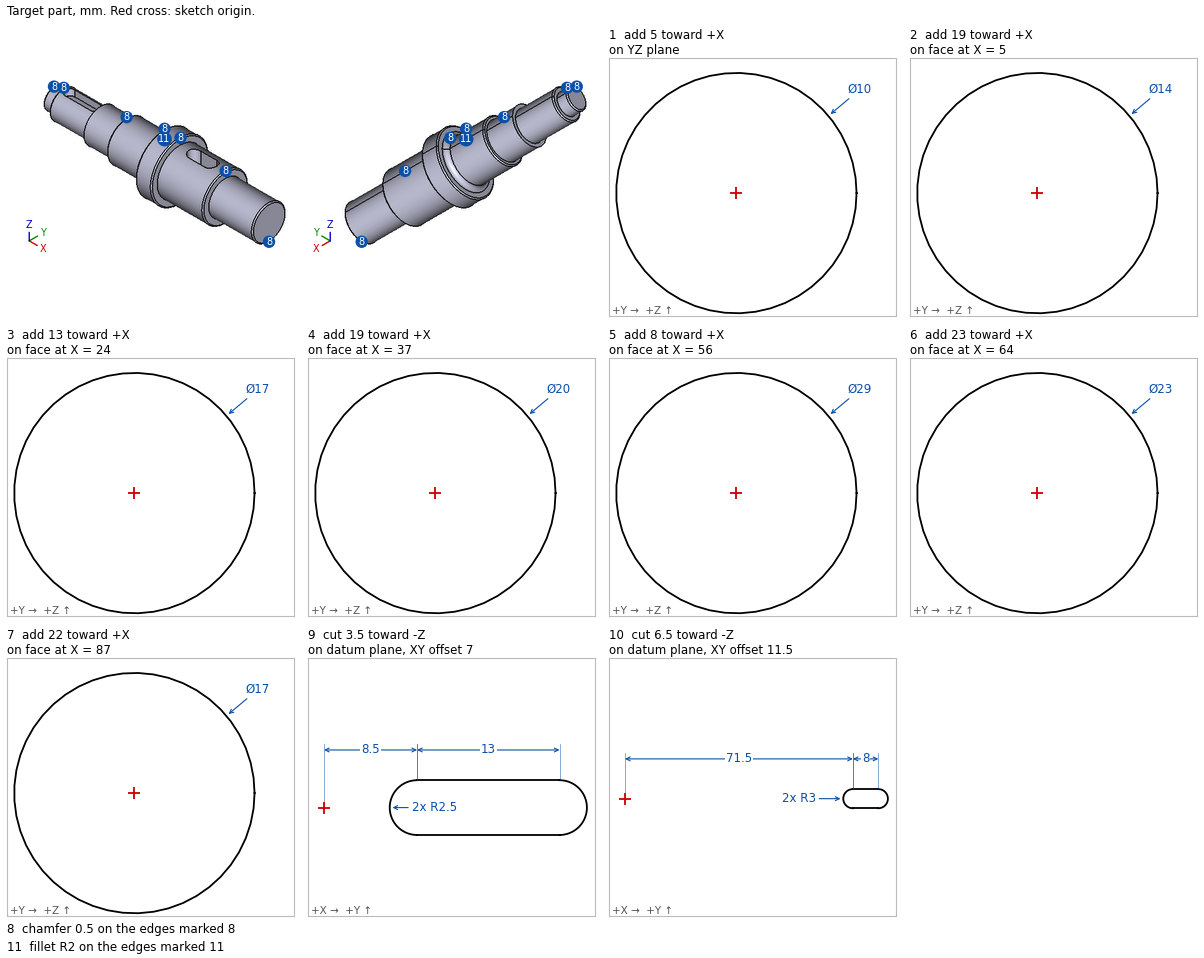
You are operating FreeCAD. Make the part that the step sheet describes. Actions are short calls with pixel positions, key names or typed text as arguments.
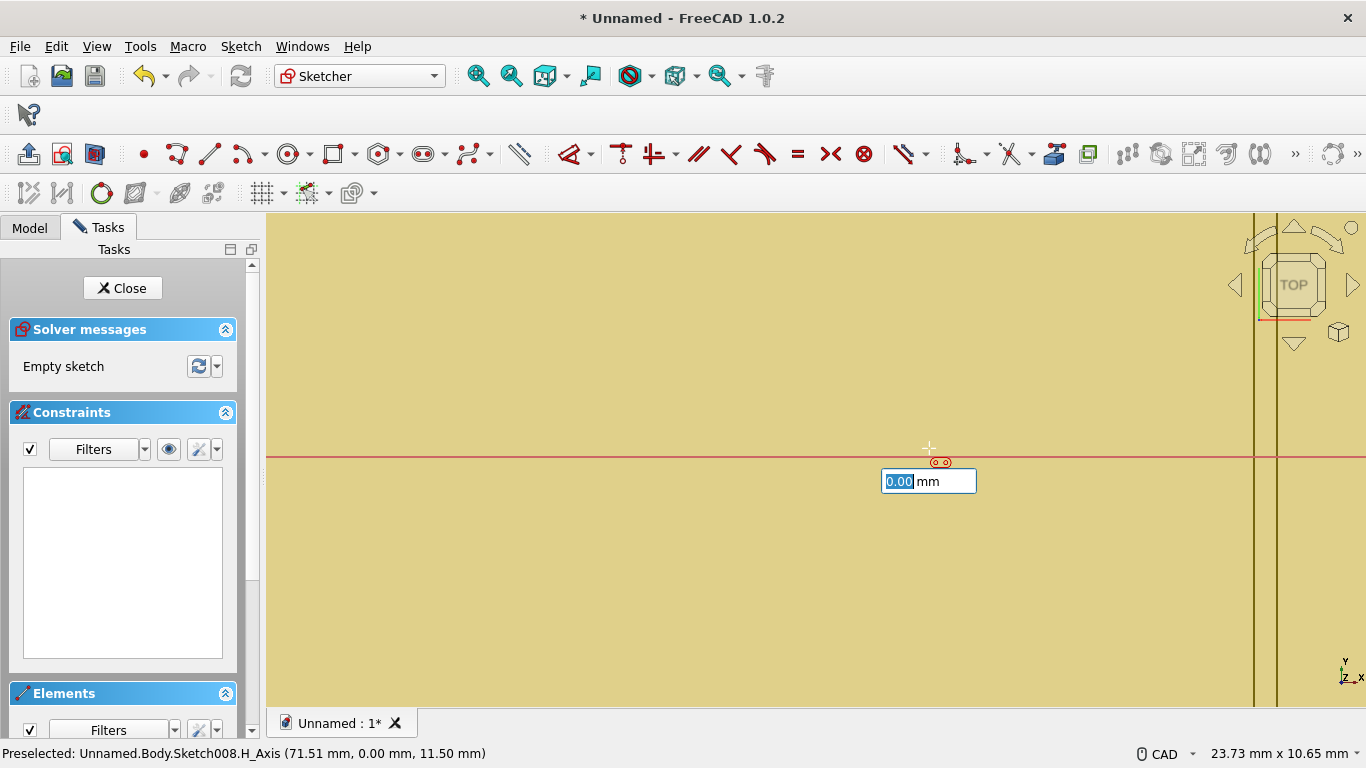
click(744, 317)
key(Escape)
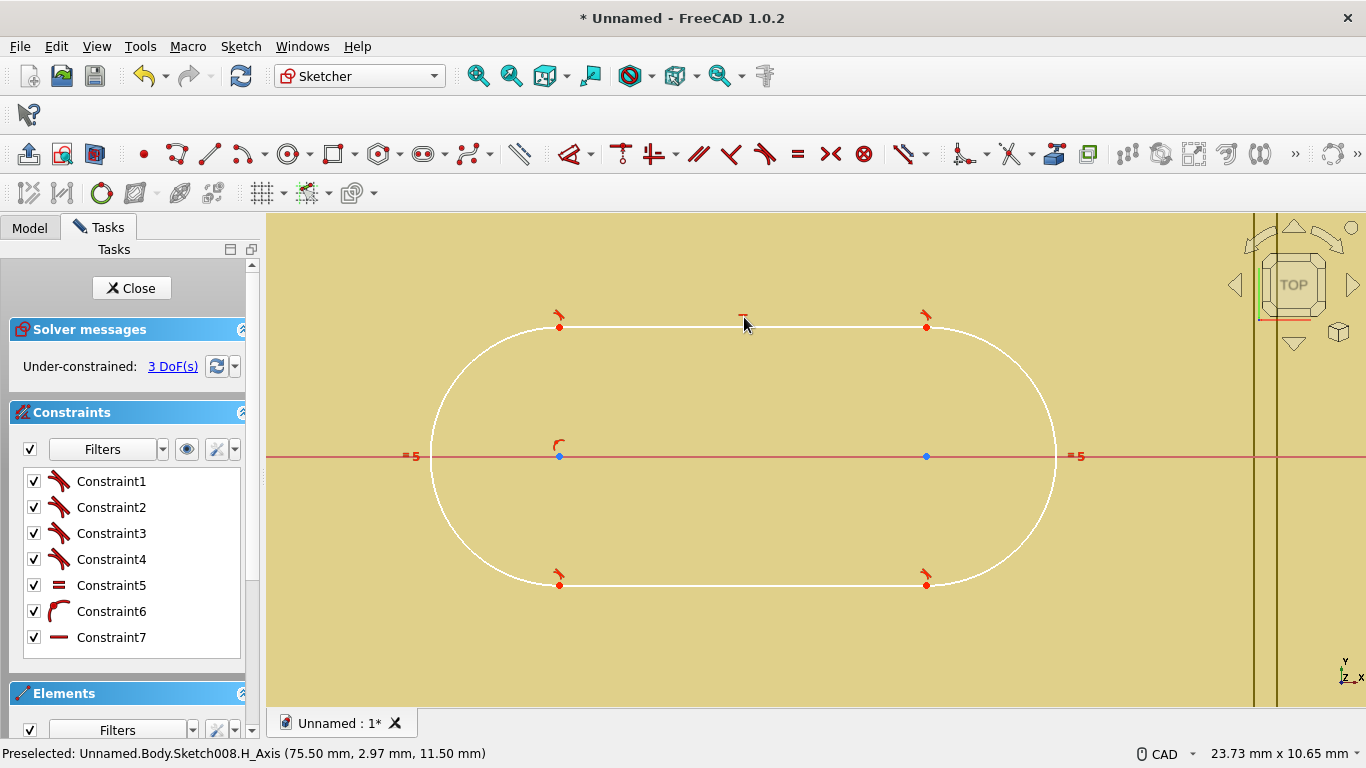
click(568, 154)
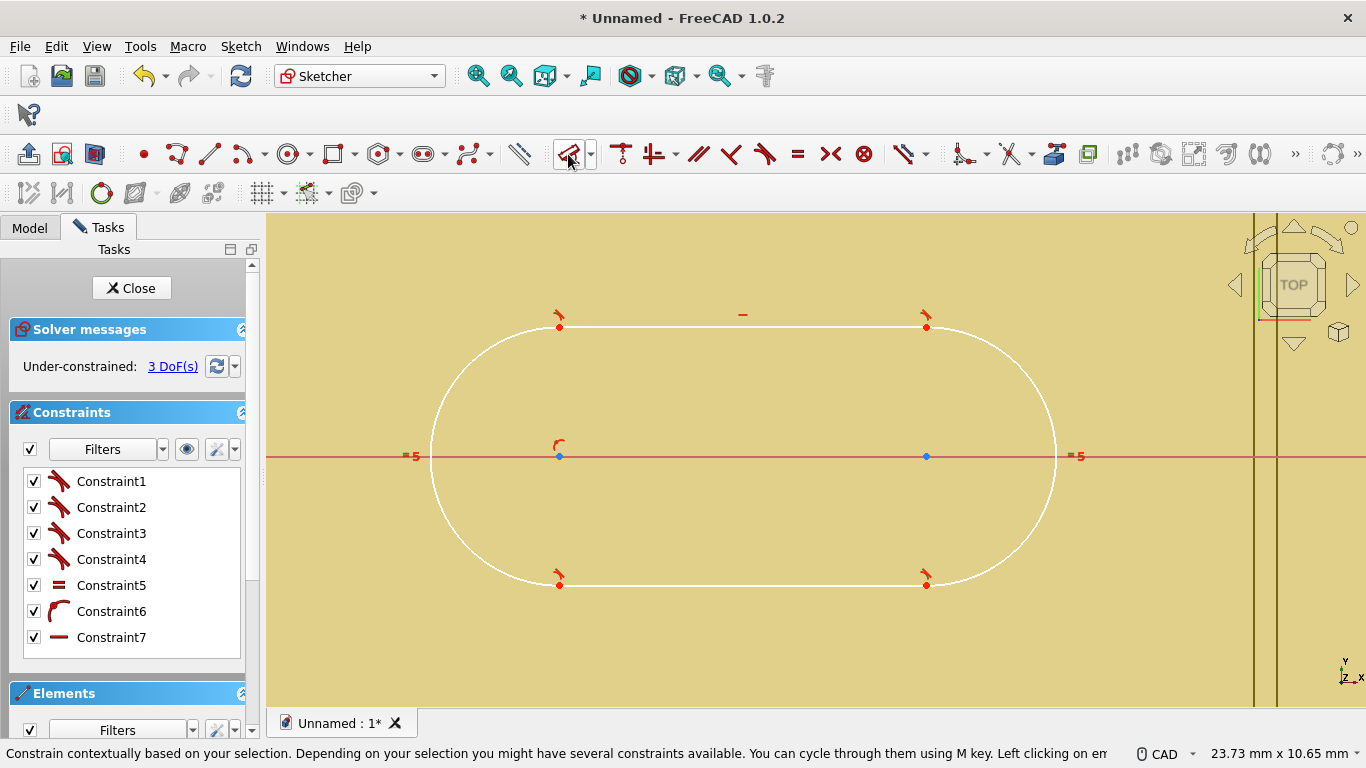
click(455, 381)
click(429, 362)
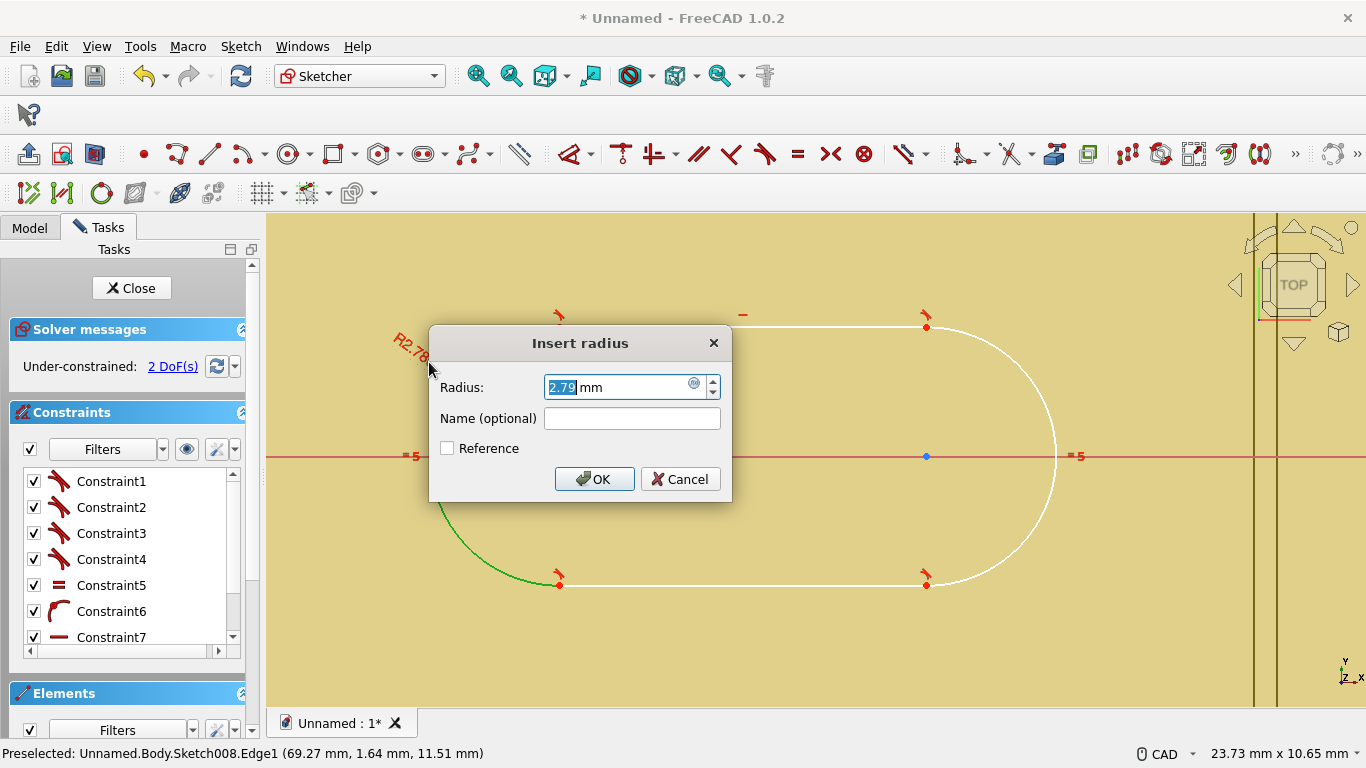
text(3)
key(Return)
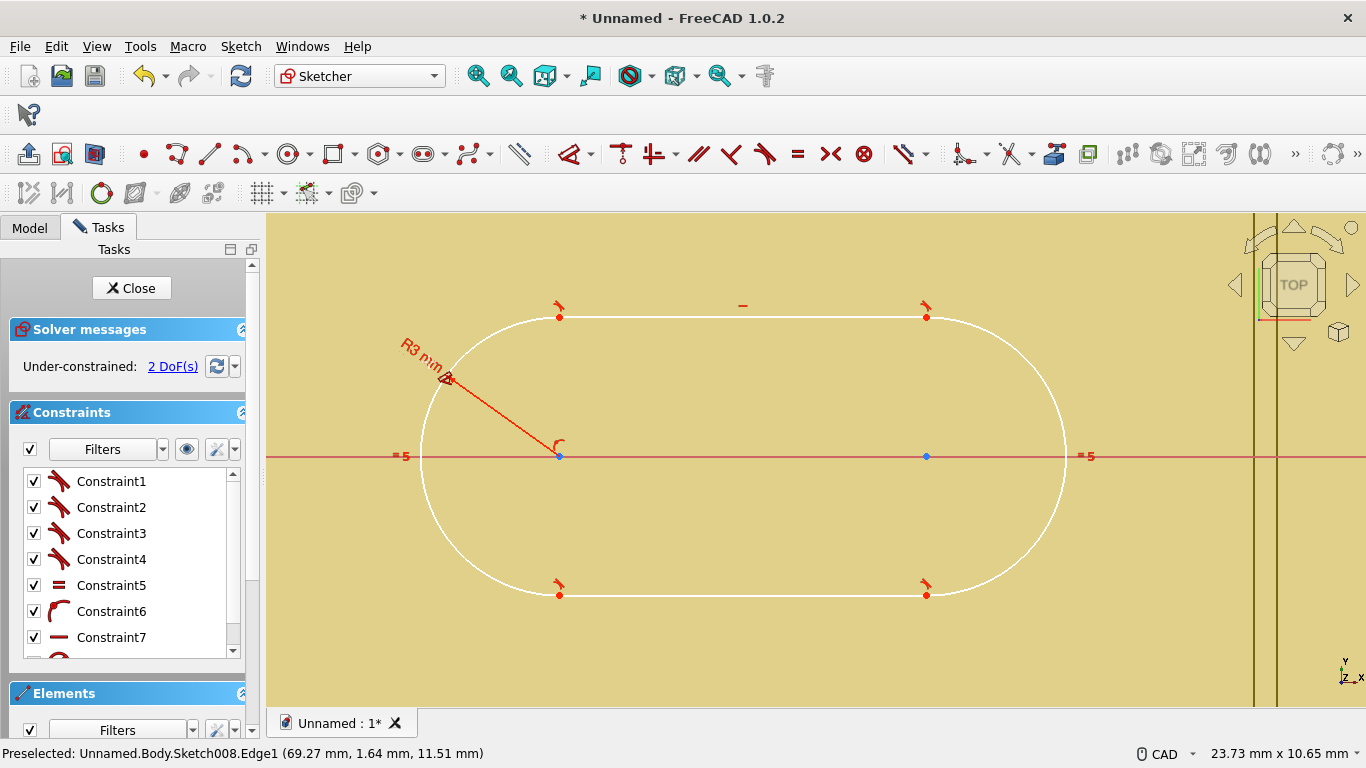
click(670, 317)
click(743, 283)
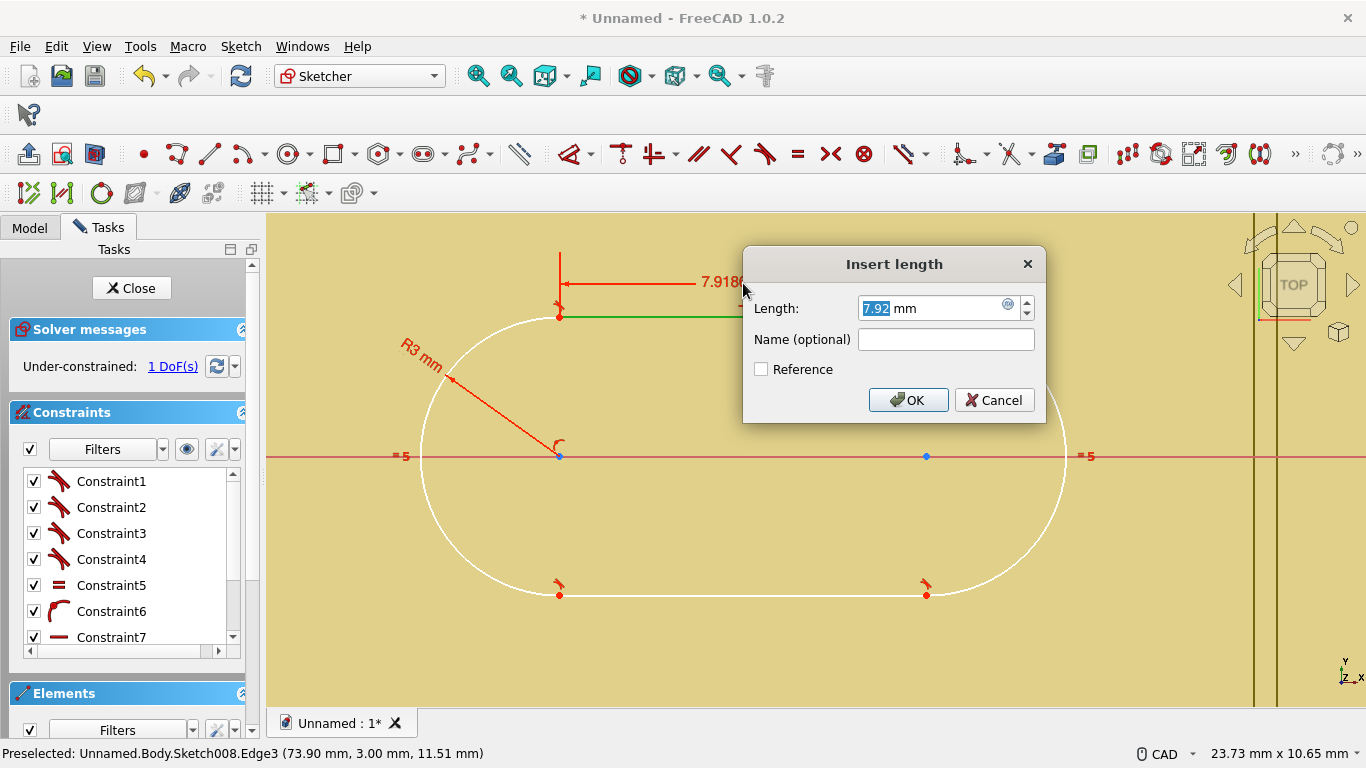
text(8)
key(Return)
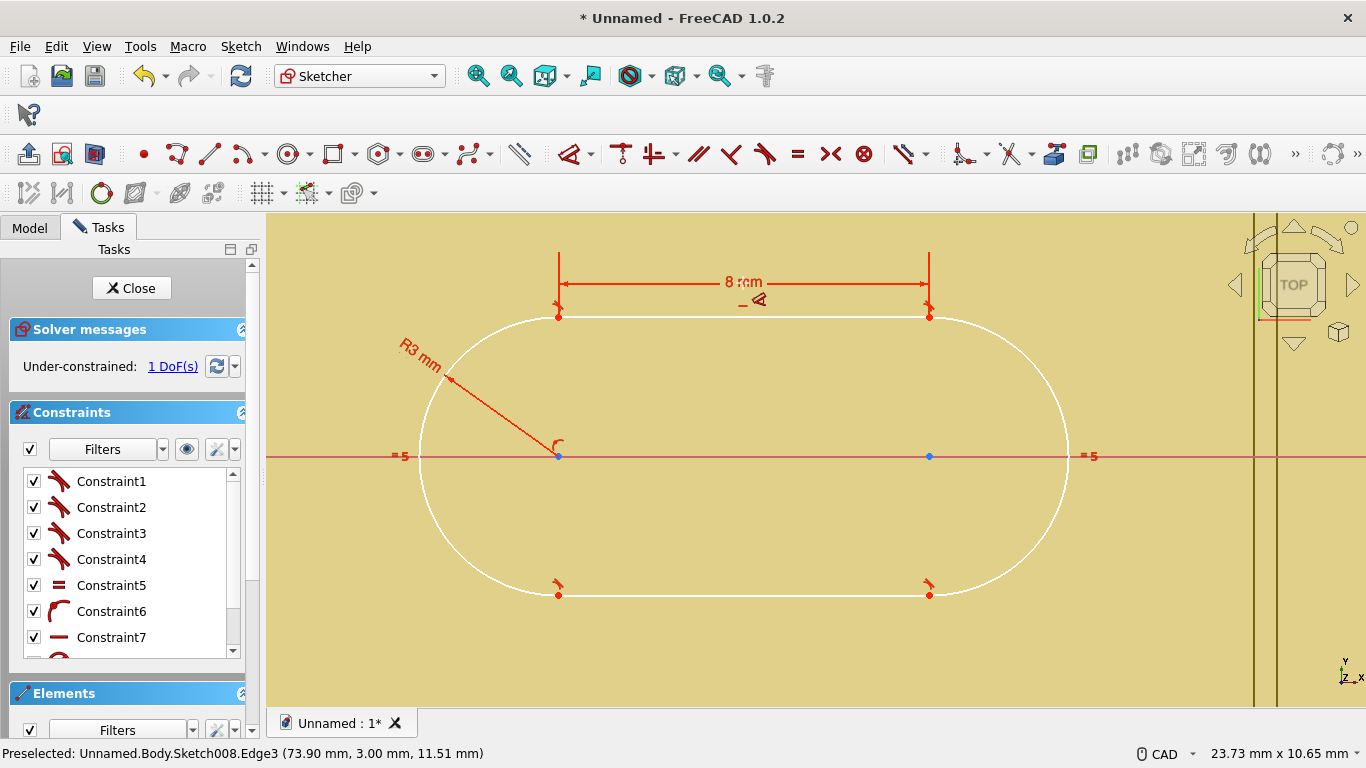
click(559, 317)
click(426, 283)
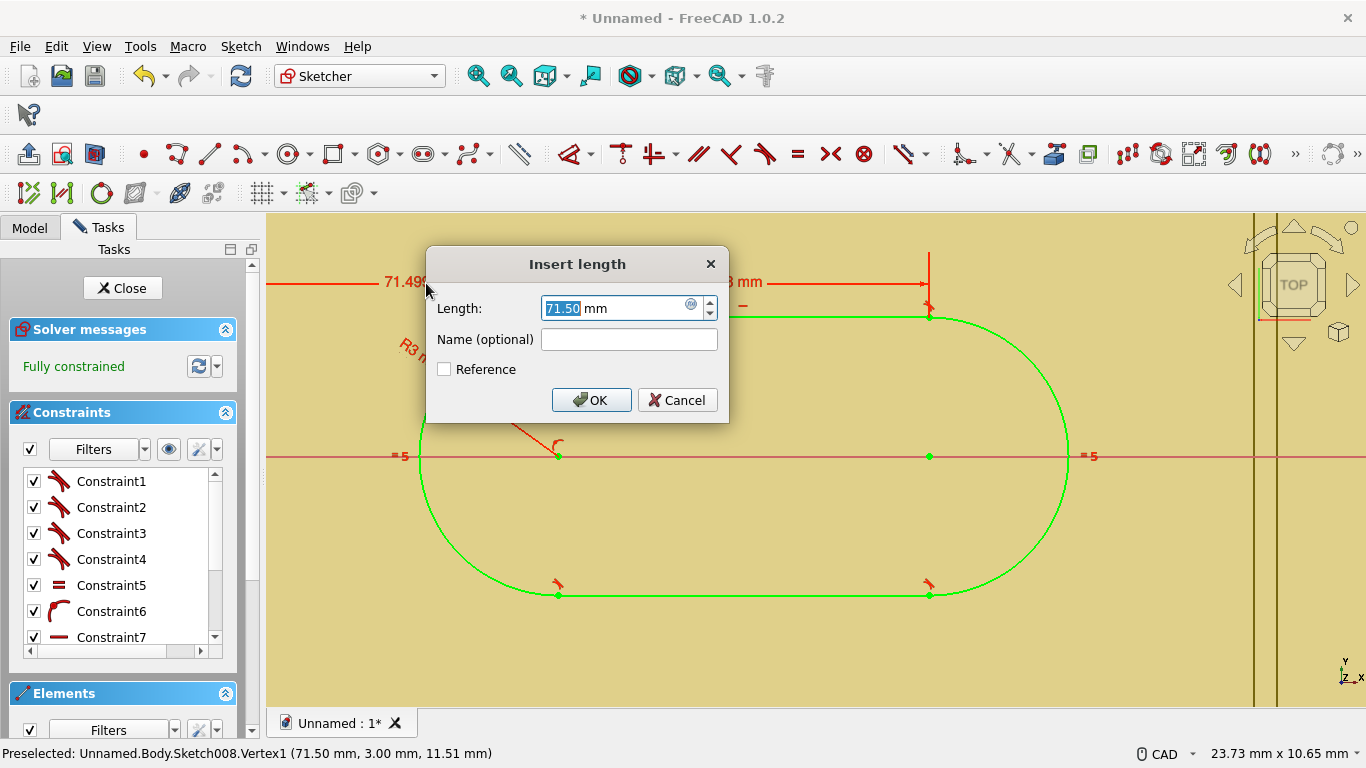
text(71.5)
key(Return)
key(Escape)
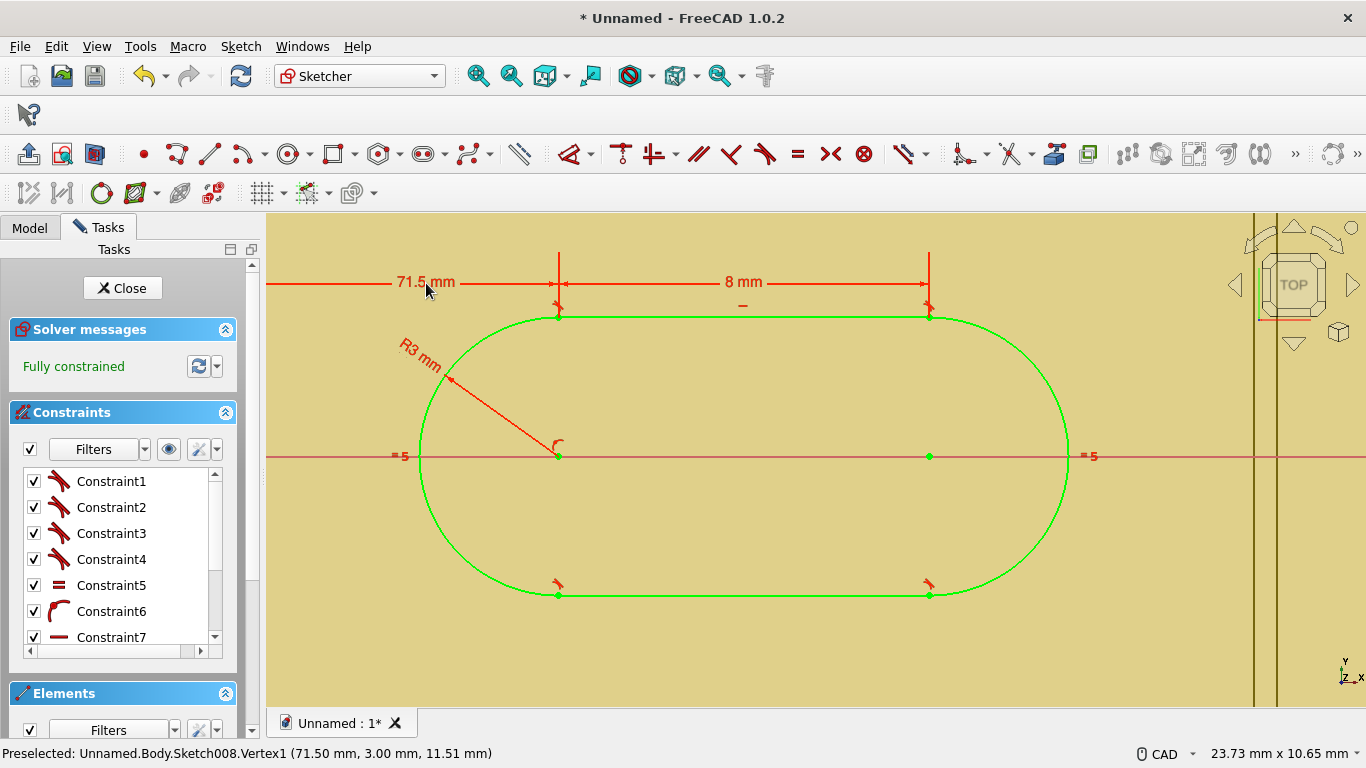
click(123, 288)